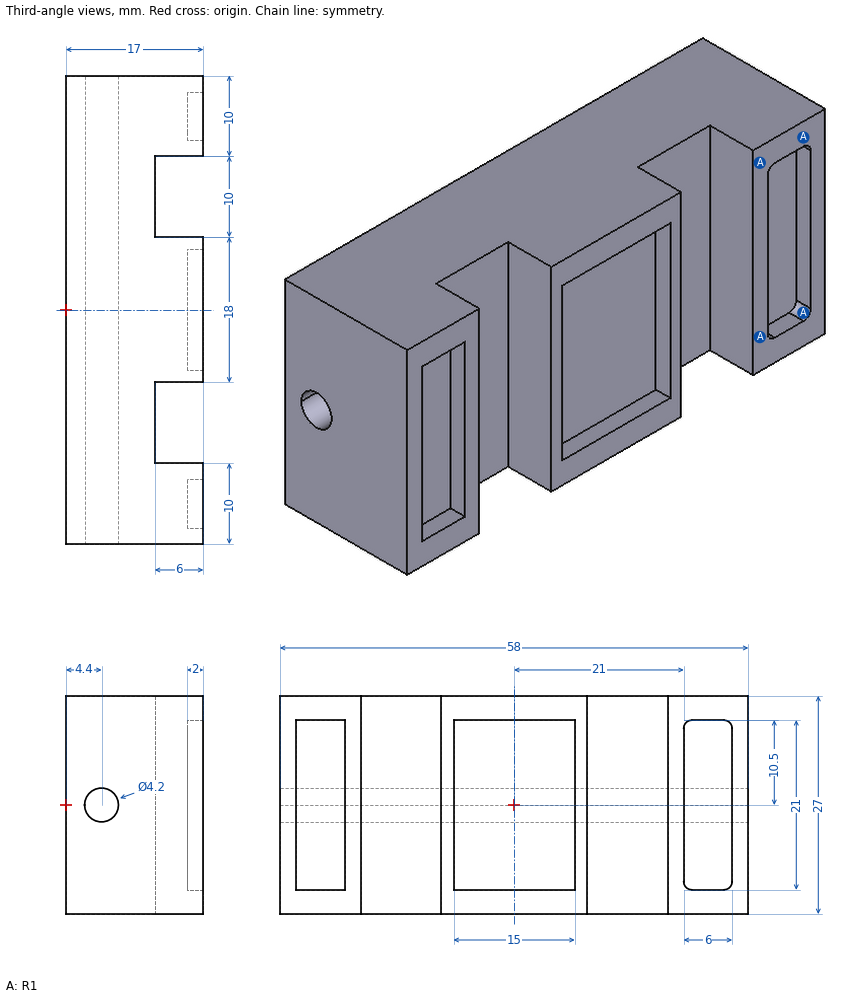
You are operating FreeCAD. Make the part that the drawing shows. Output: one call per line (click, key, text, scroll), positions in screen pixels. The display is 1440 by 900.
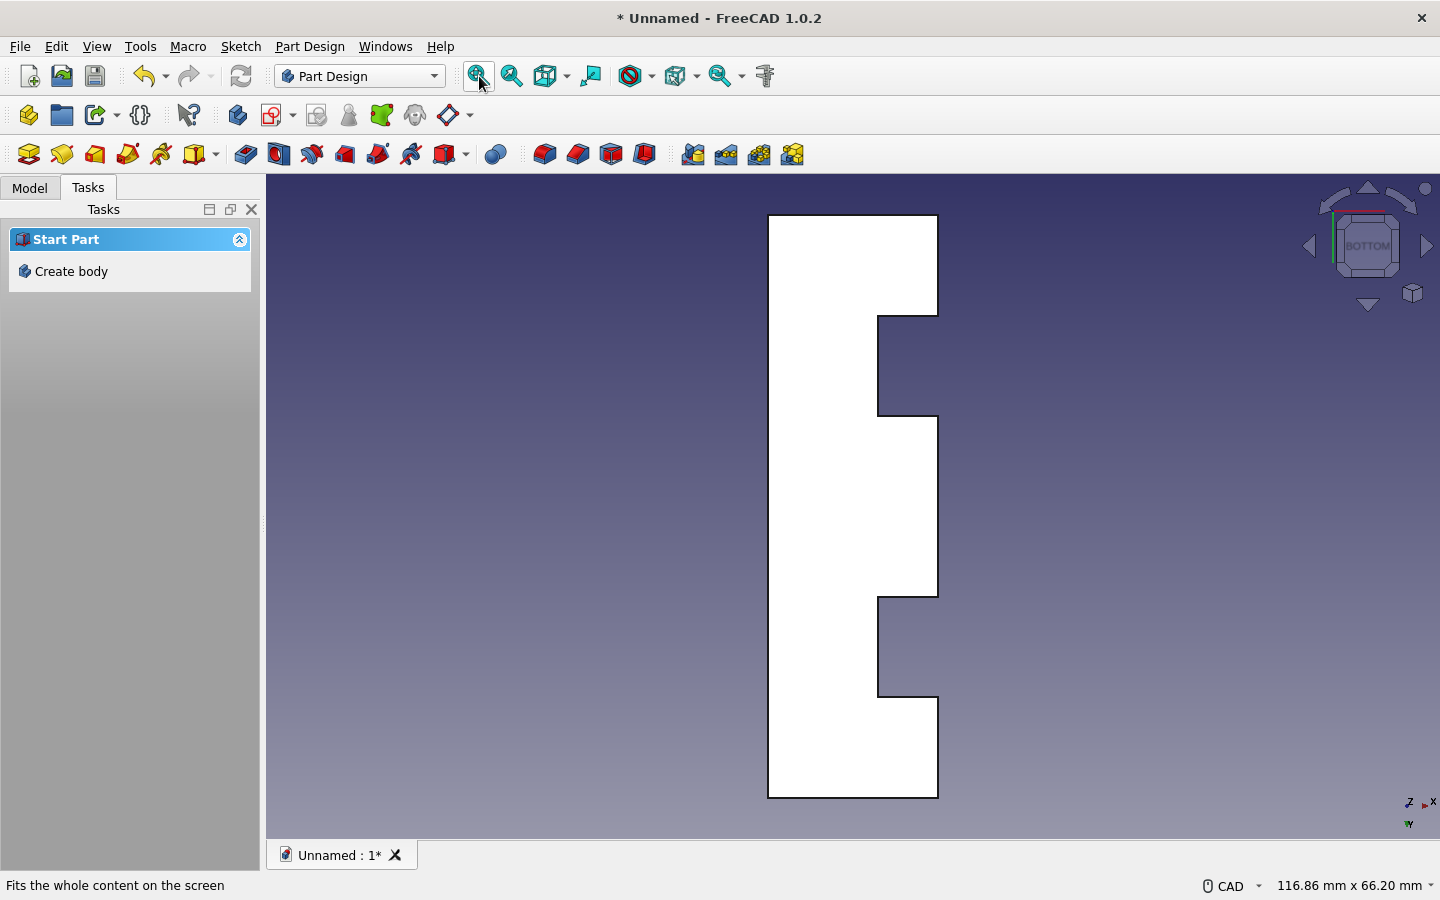
key(4)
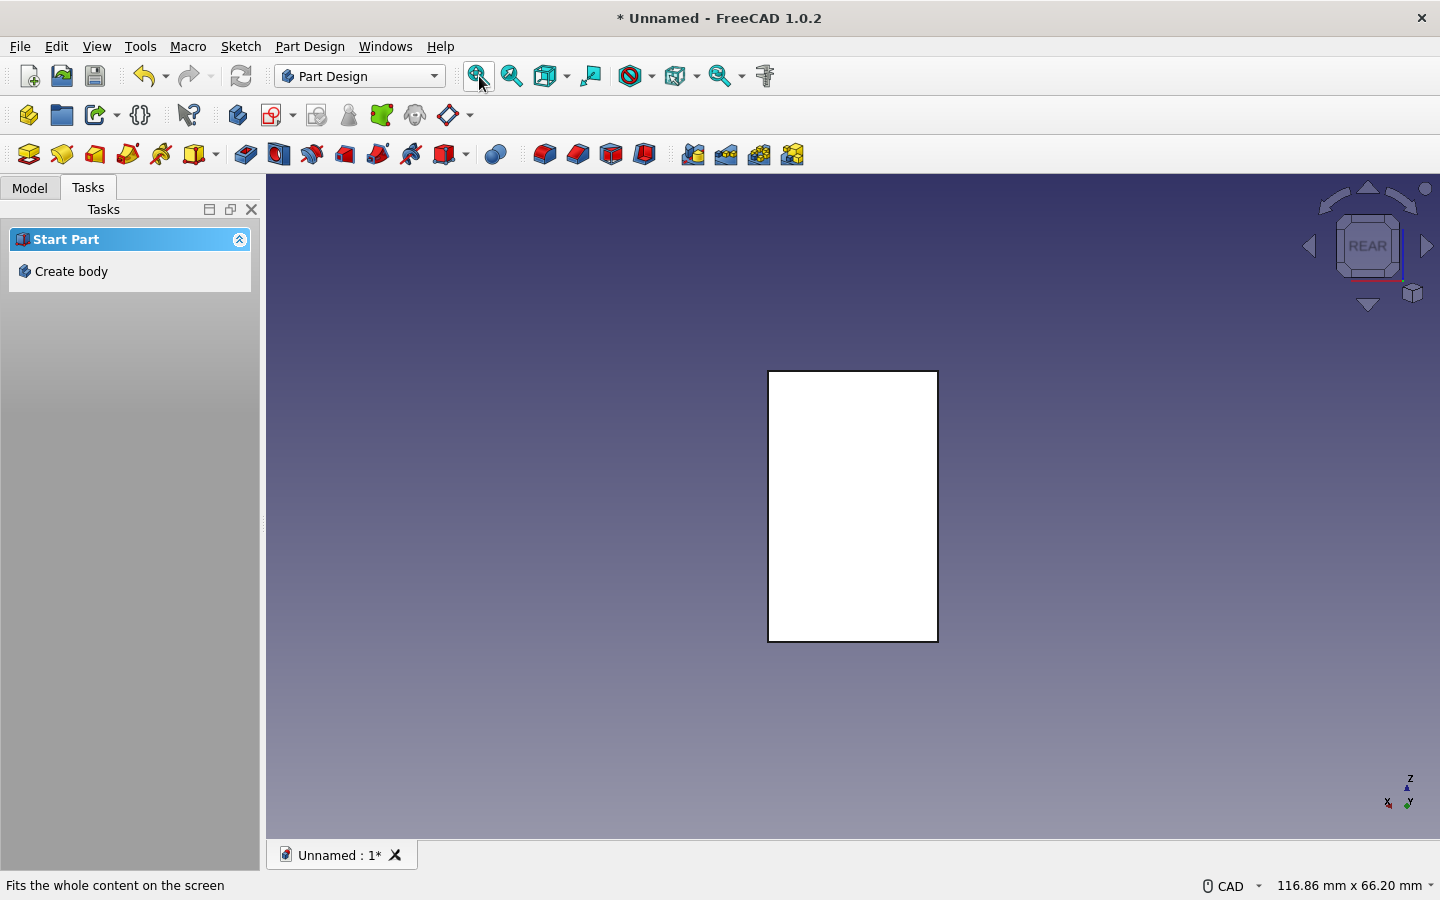
key(v)
key(f)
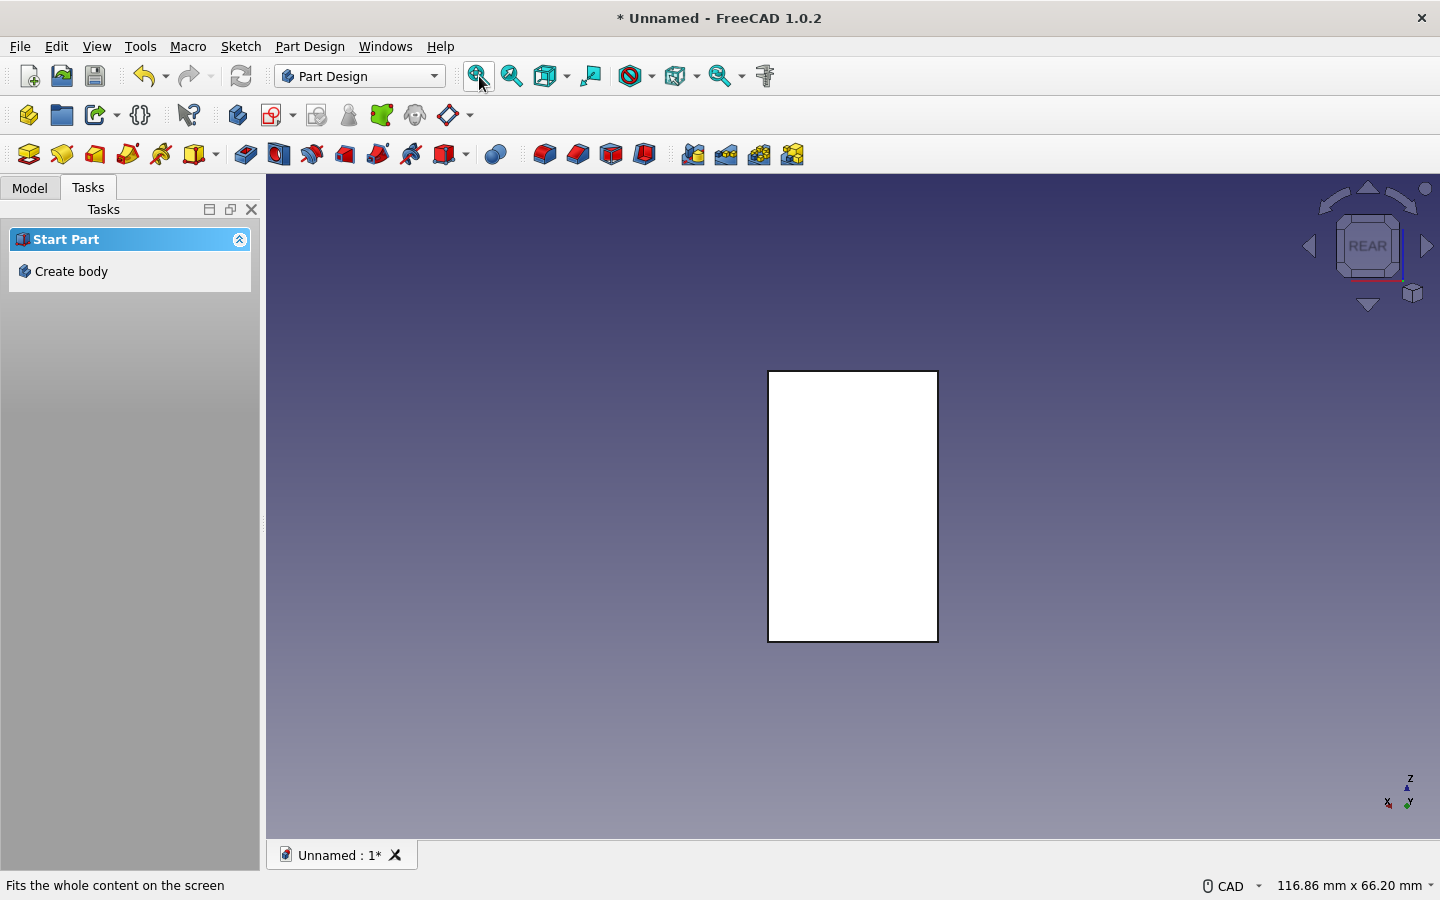
scroll(778, 611, up, 4)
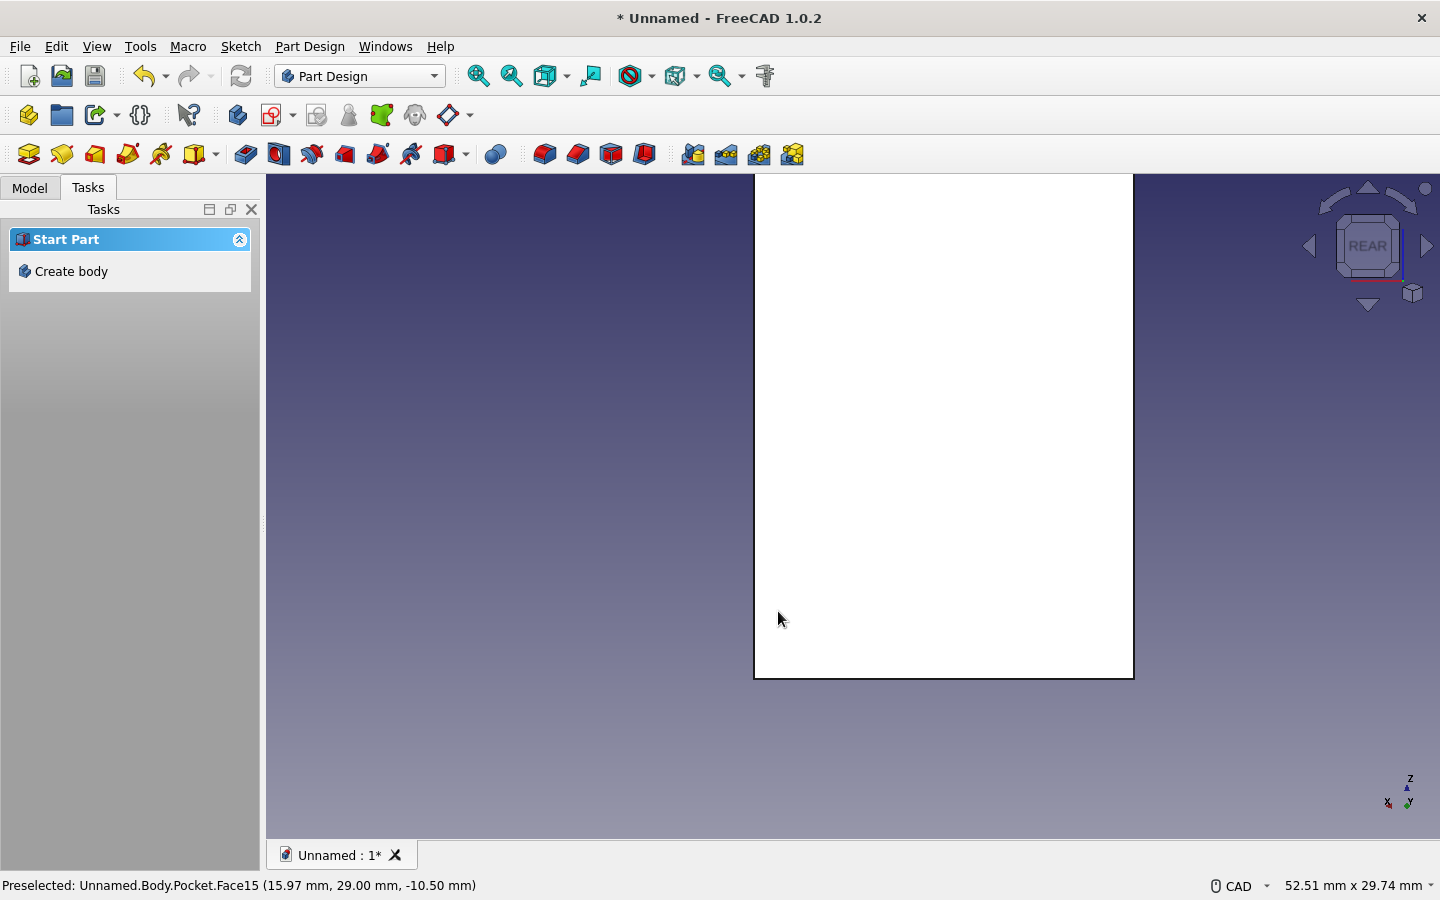
click(479, 76)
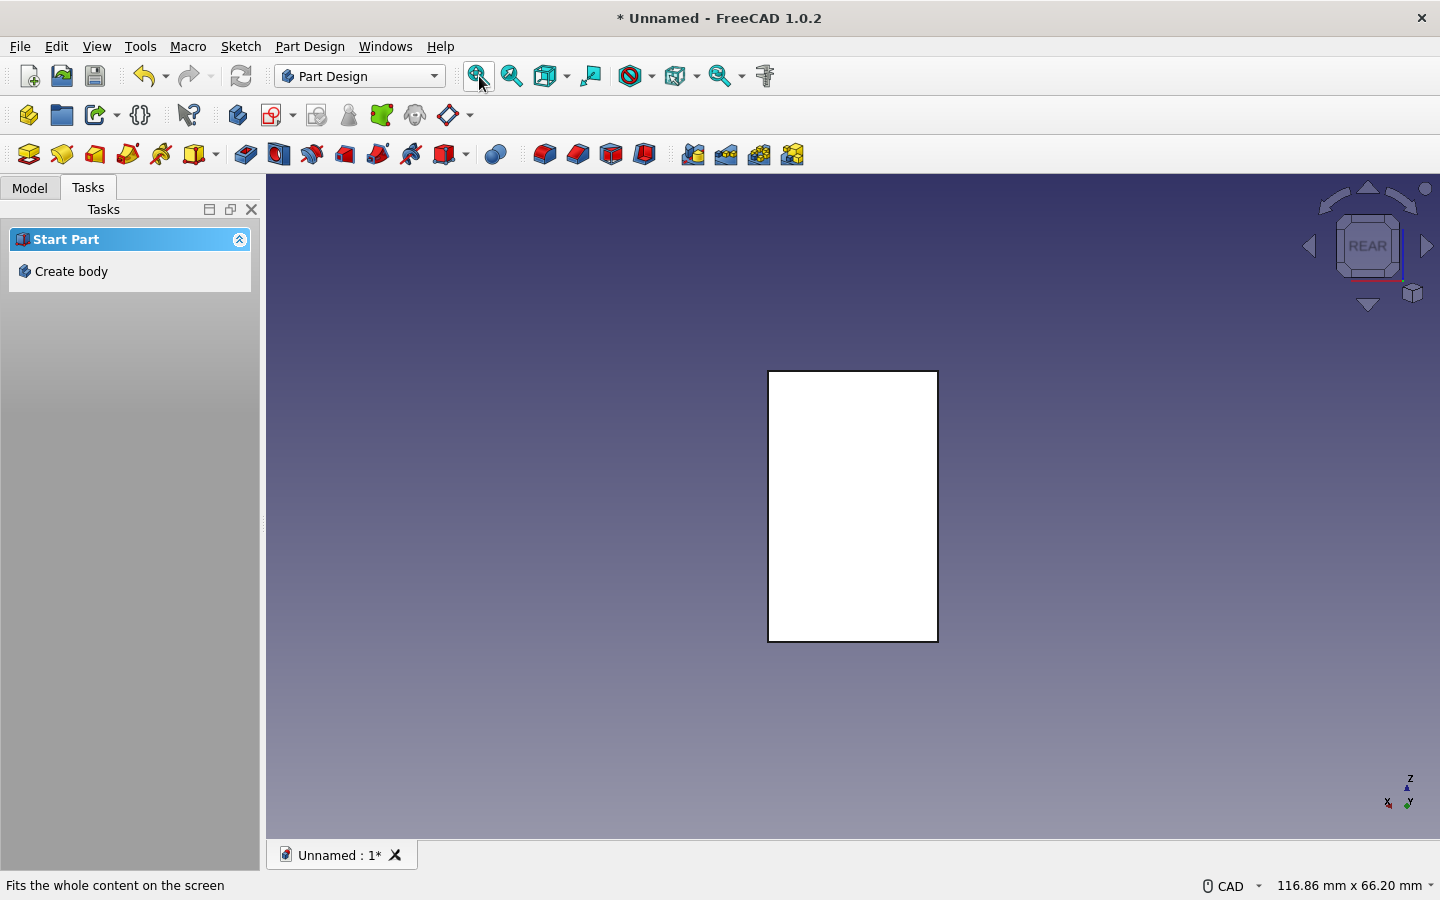
key(6)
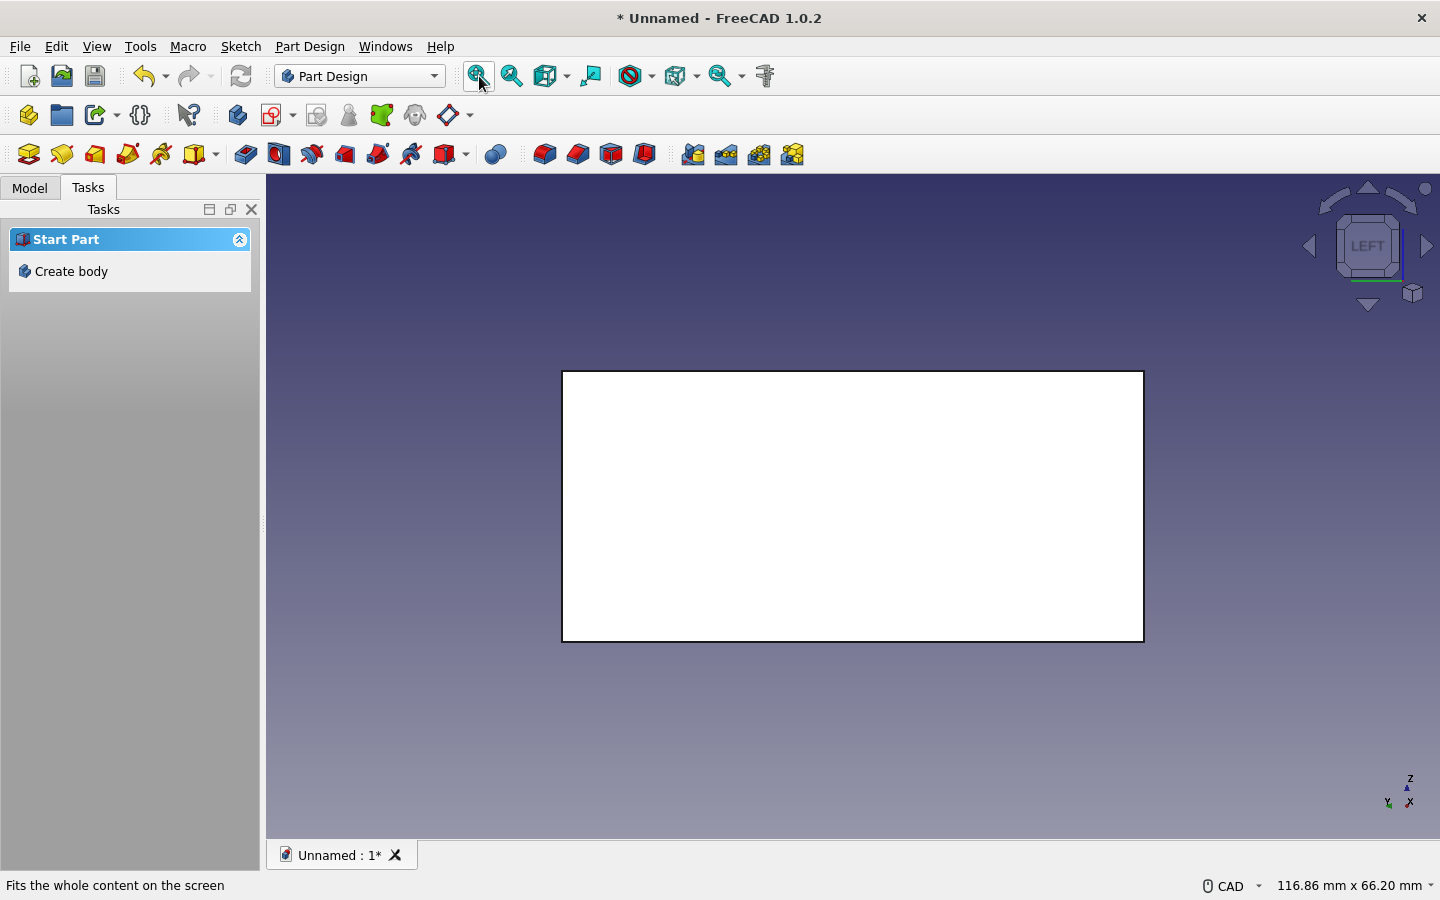
scroll(582, 611, up, 4)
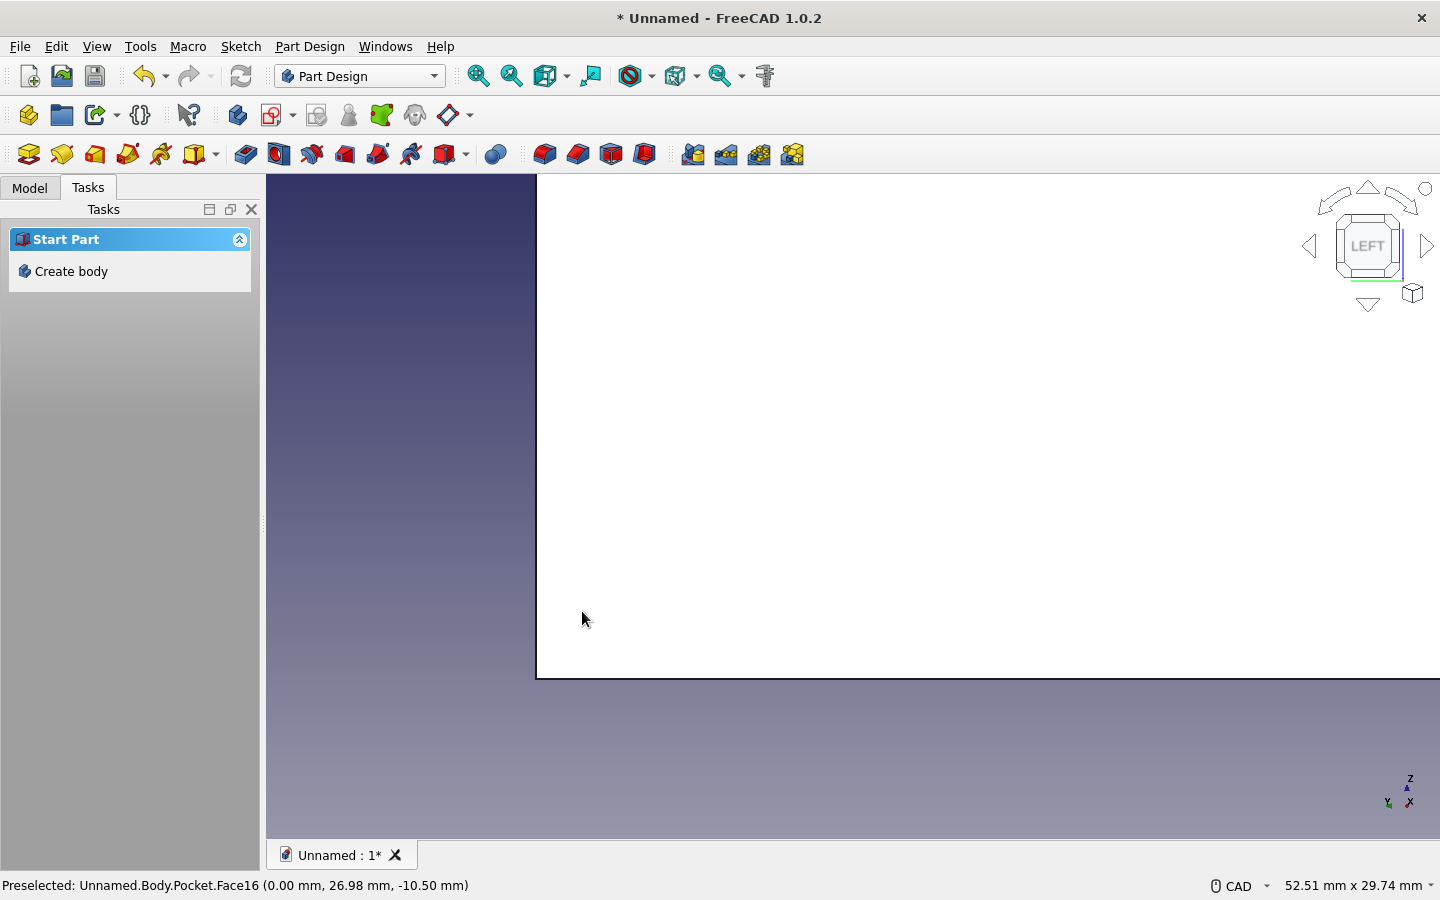
key(v)
key(f)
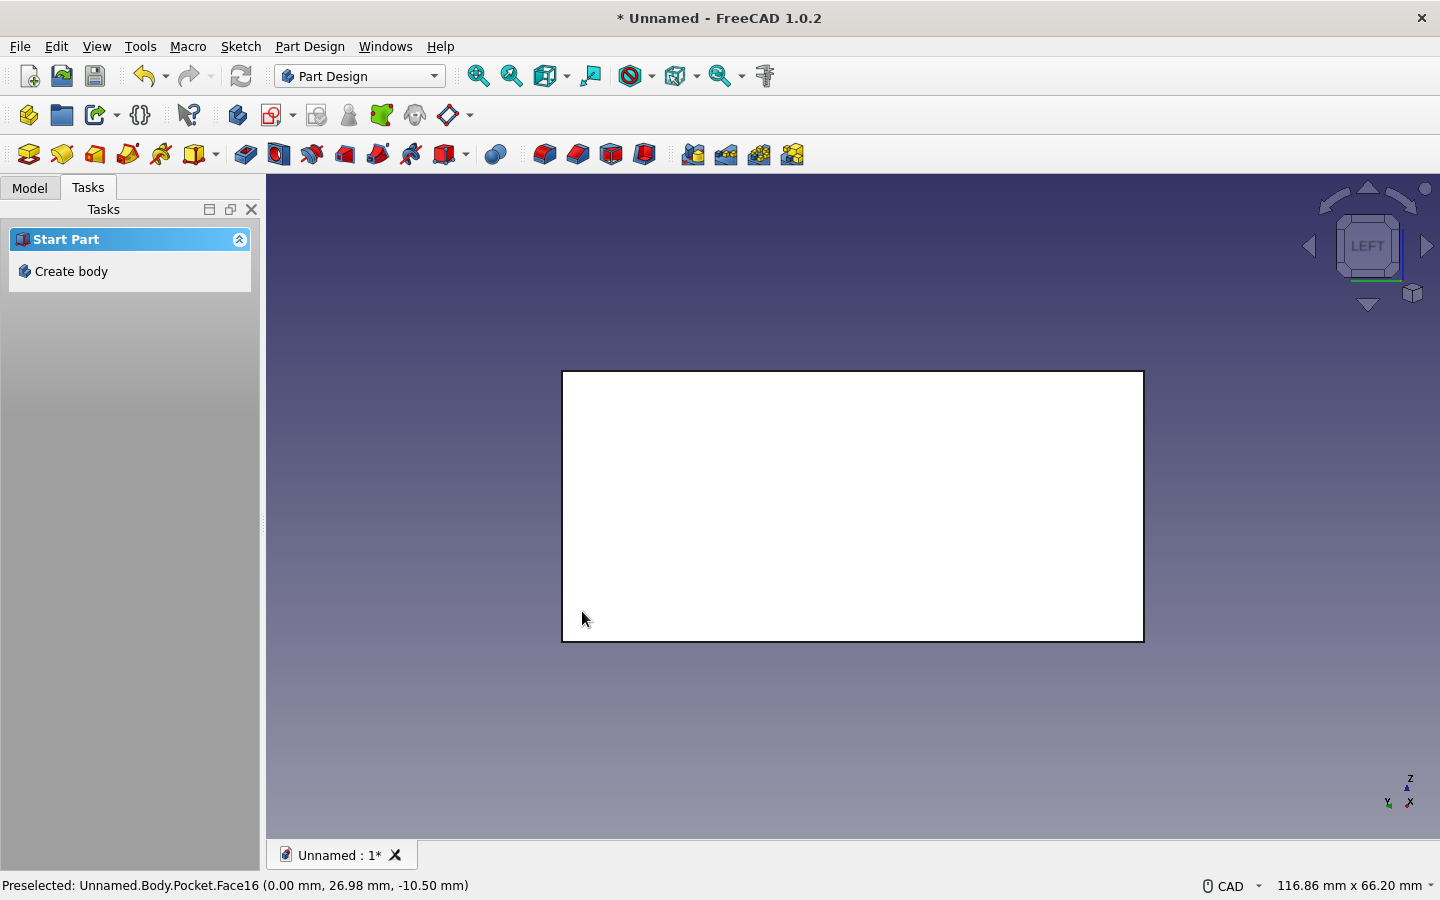
key(v)
key(3)